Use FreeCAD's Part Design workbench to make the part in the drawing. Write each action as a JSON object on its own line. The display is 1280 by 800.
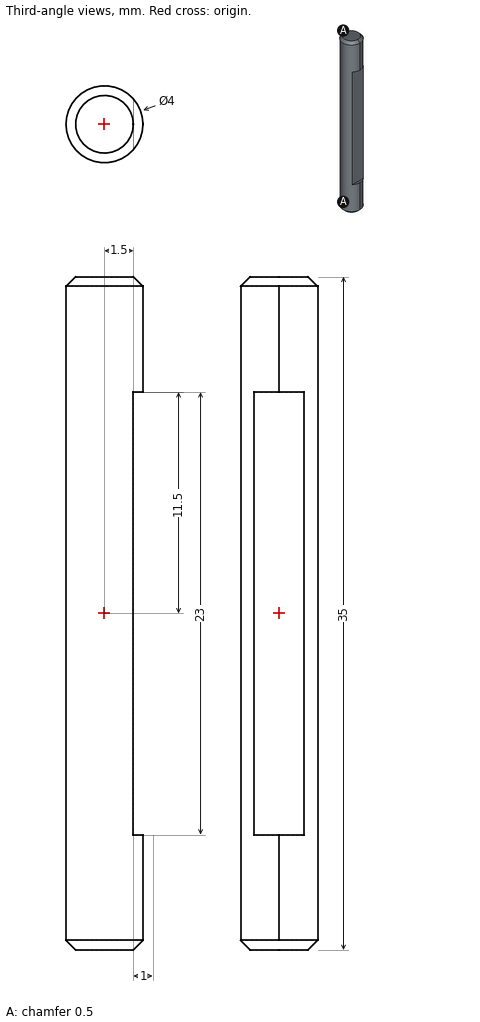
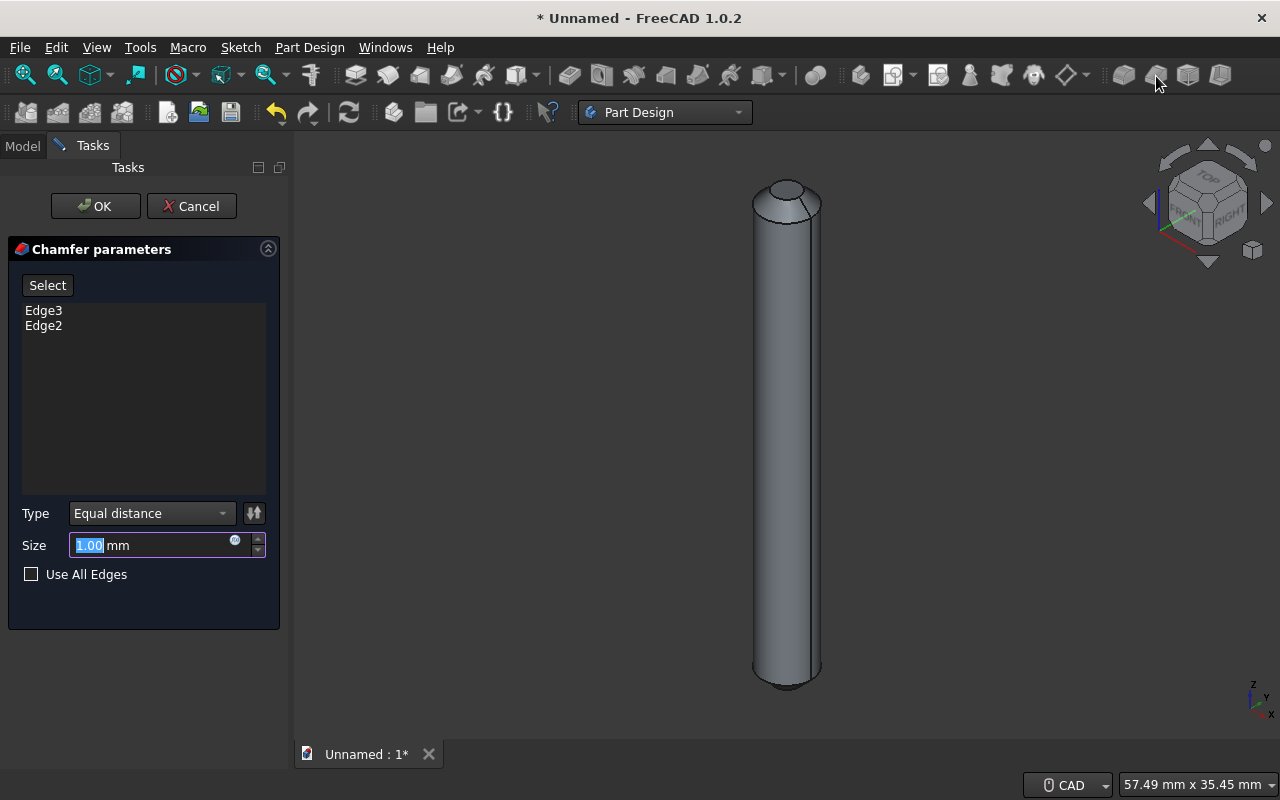
{"action": "type", "text": "0.5"}
{"action": "key", "text": "Tab"}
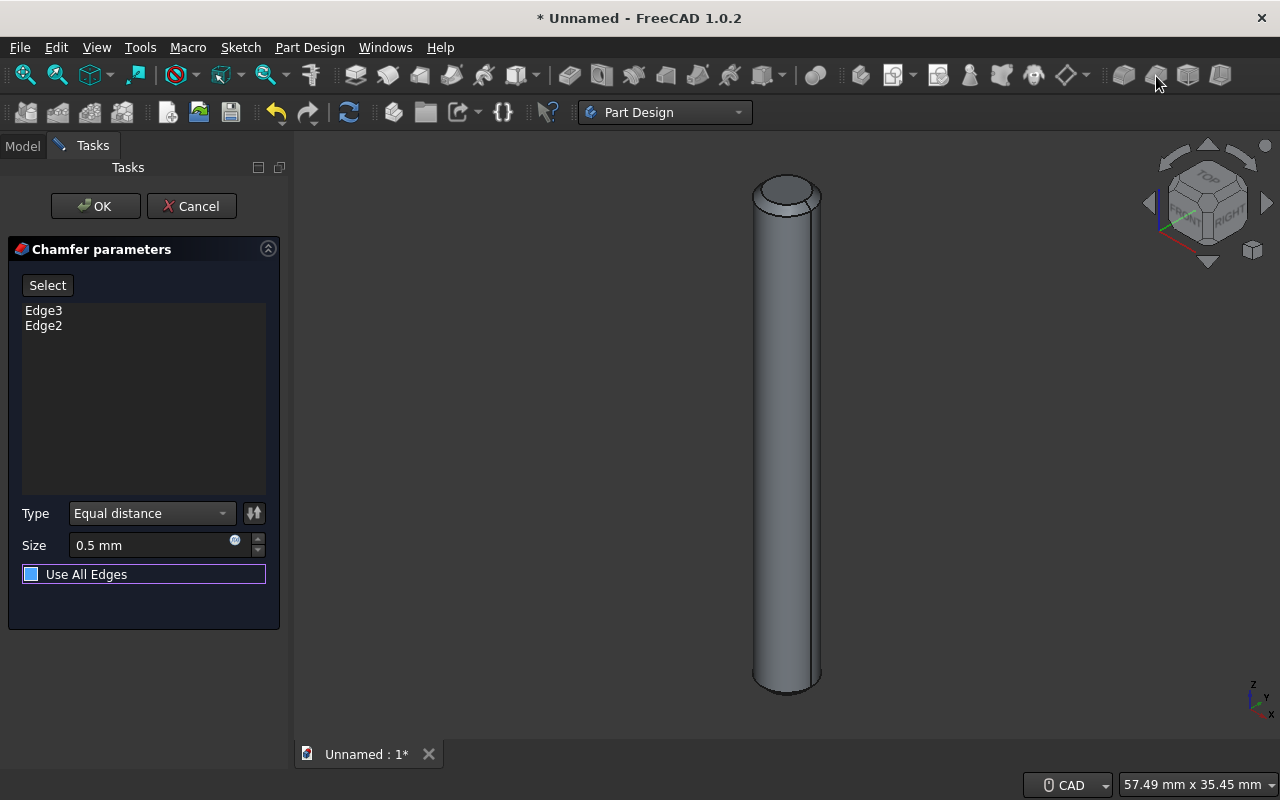
{"action": "left_click", "coordinate": [96, 206]}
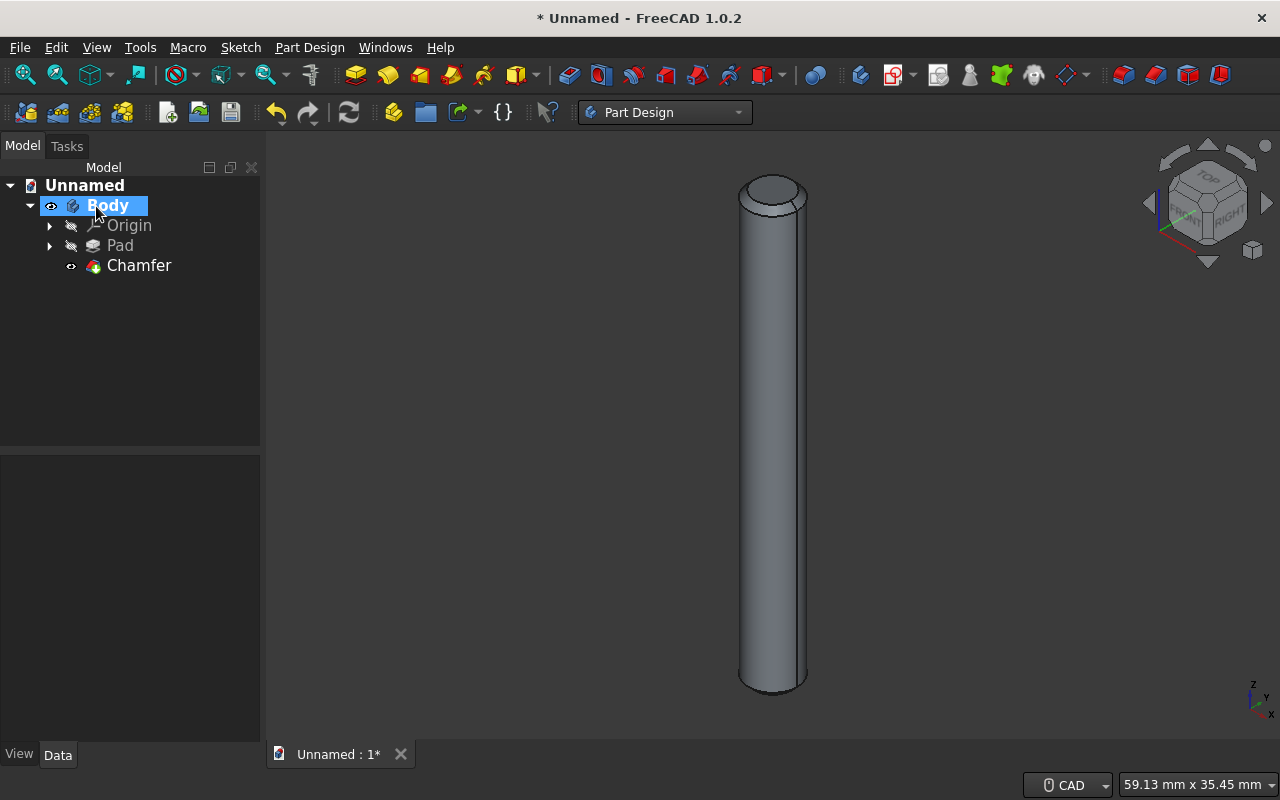
{"action": "left_click", "coordinate": [894, 76]}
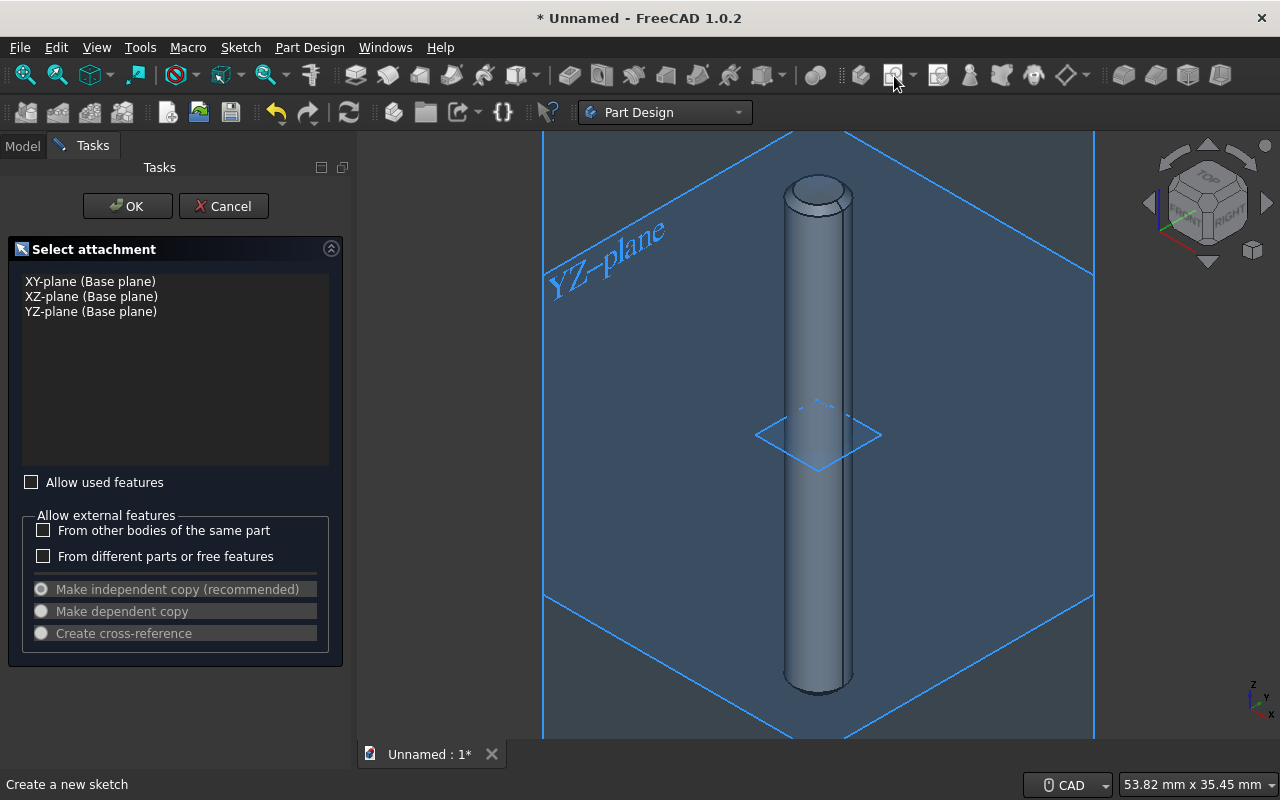
{"action": "left_click", "coordinate": [82, 296]}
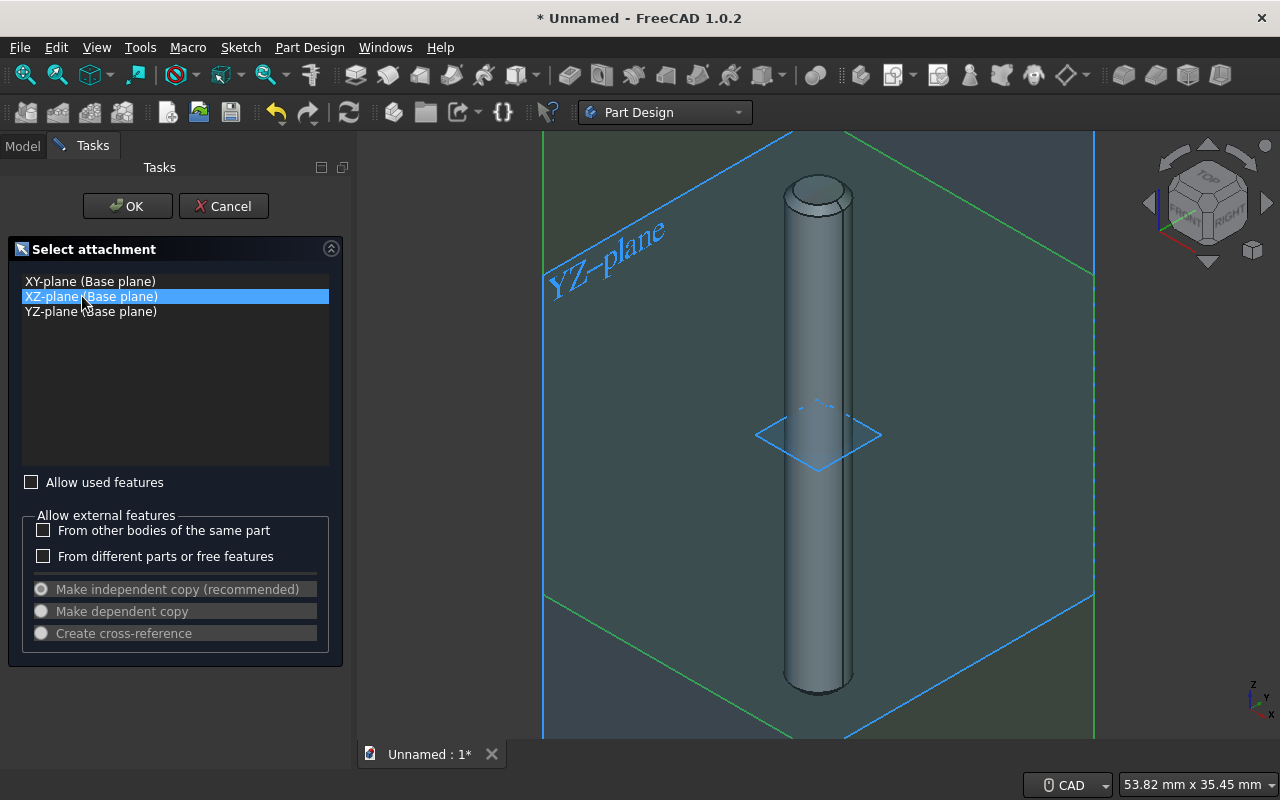
{"action": "left_click", "coordinate": [128, 206]}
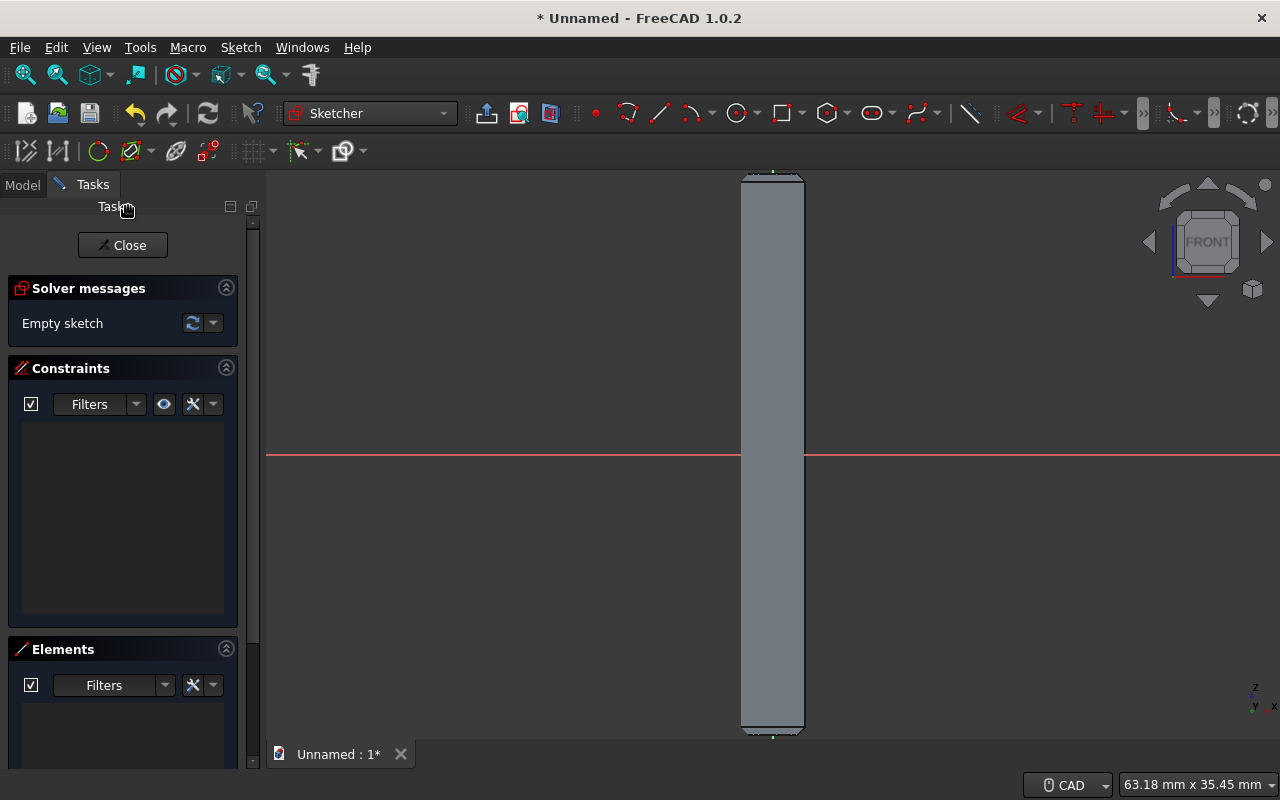
{"action": "key", "text": "q s"}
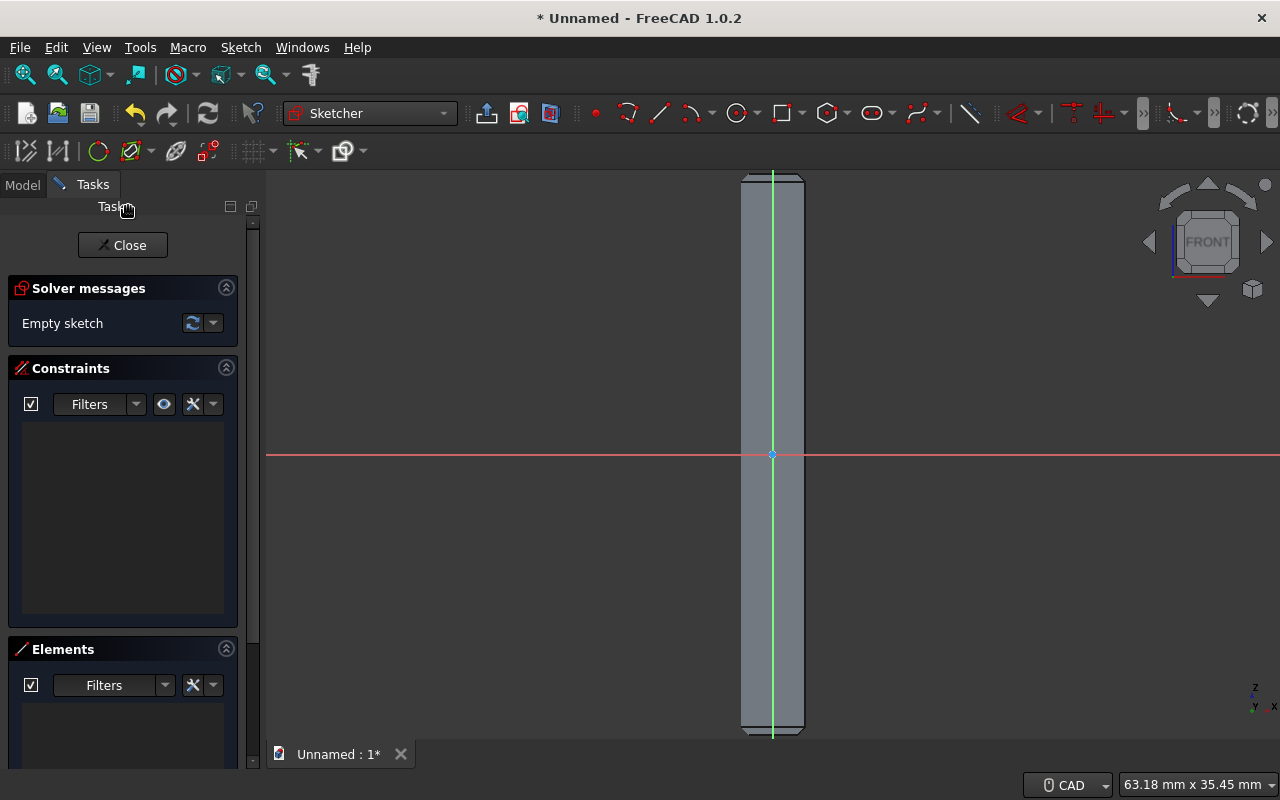
{"action": "left_click", "coordinate": [782, 114]}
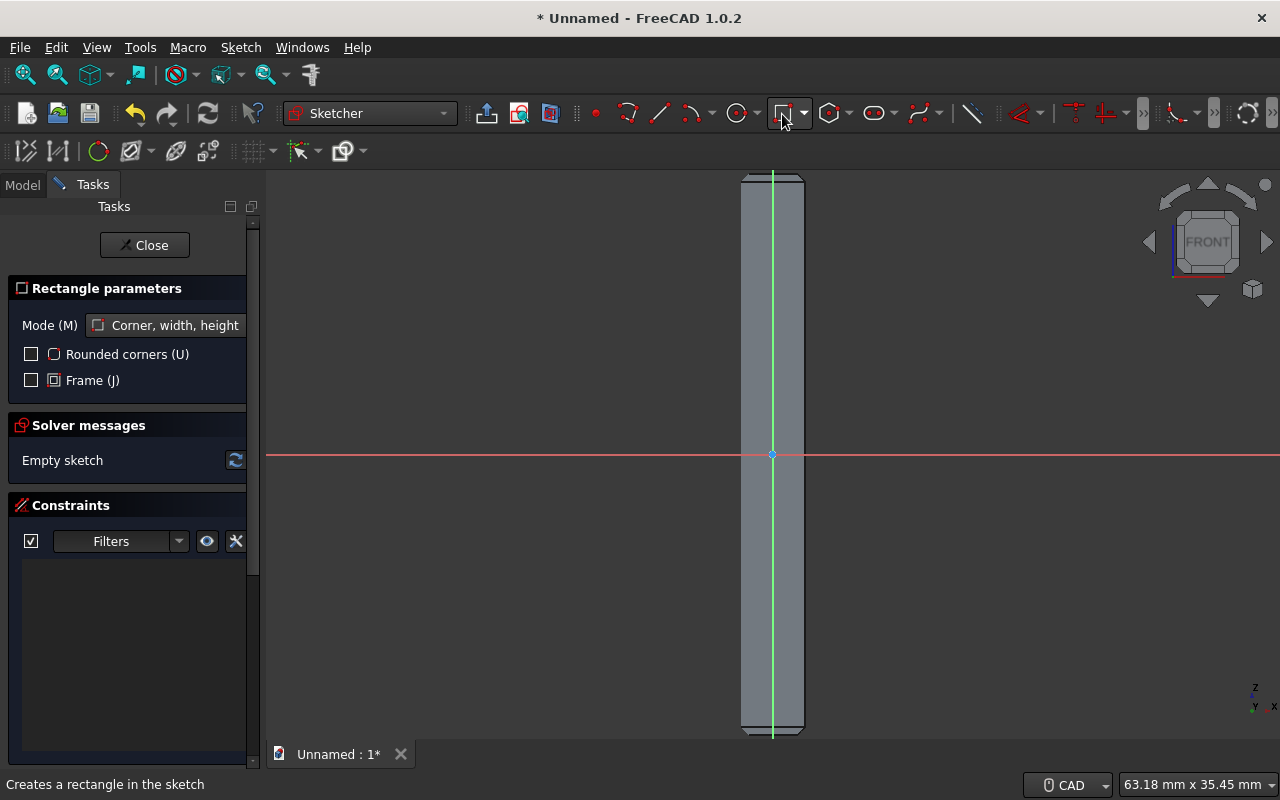
{"action": "left_click", "coordinate": [797, 270]}
{"action": "left_click", "coordinate": [813, 639]}
{"action": "key", "text": "Escape"}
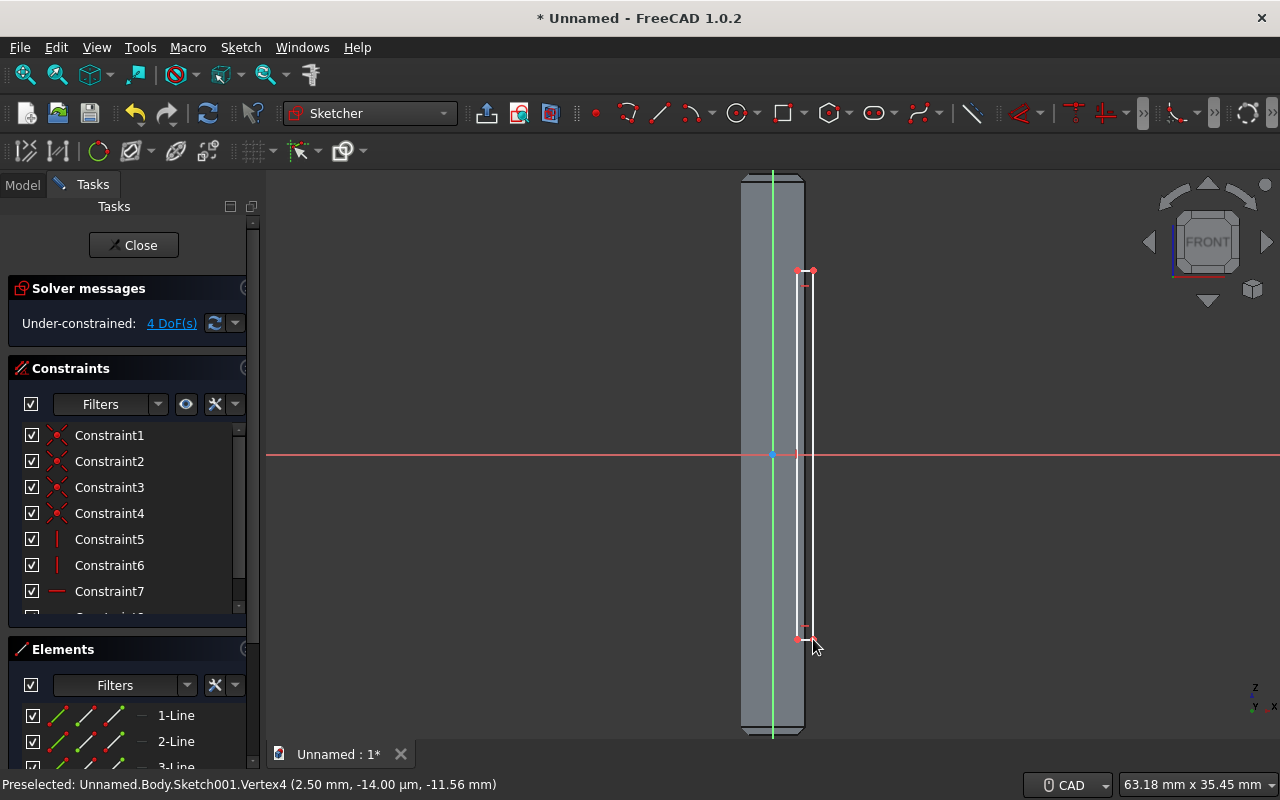
{"action": "key", "text": "d"}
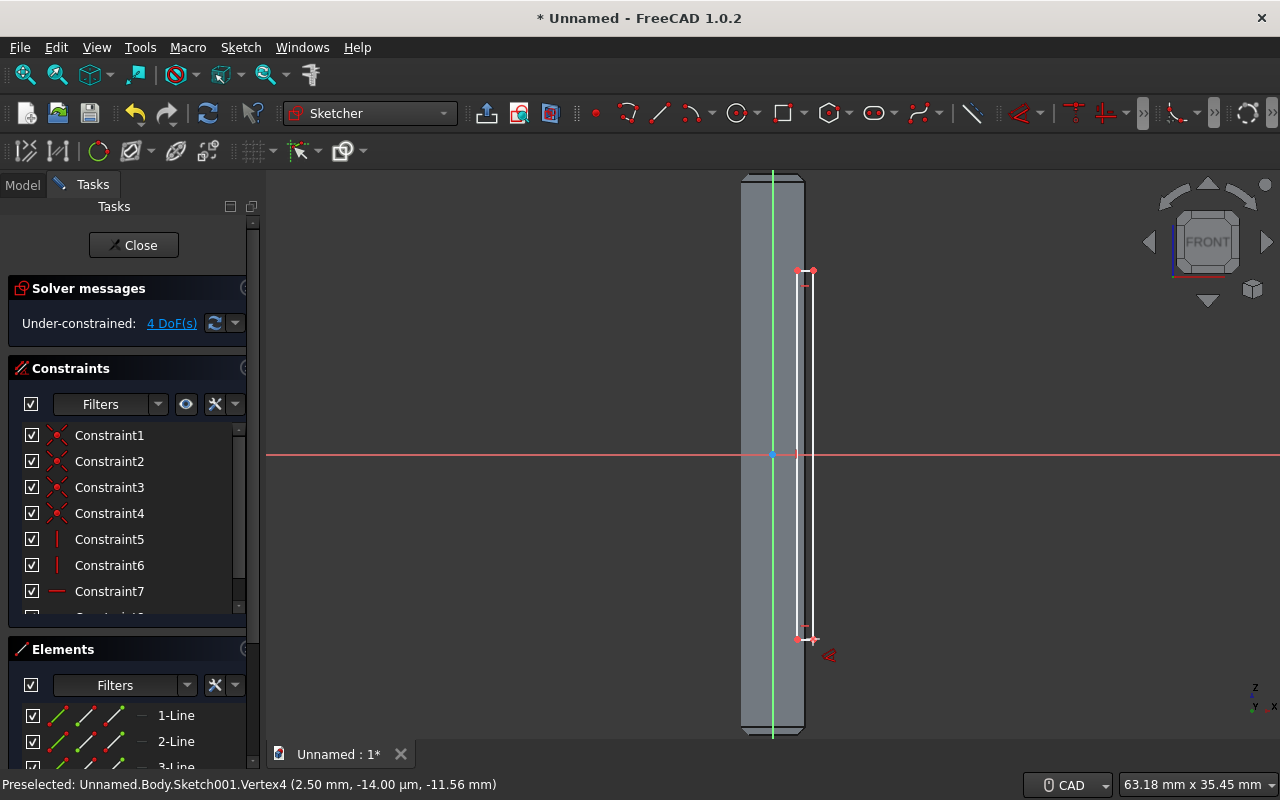
{"action": "scroll", "coordinate": [805, 640], "scroll_direction": "up", "scroll_amount": 5}